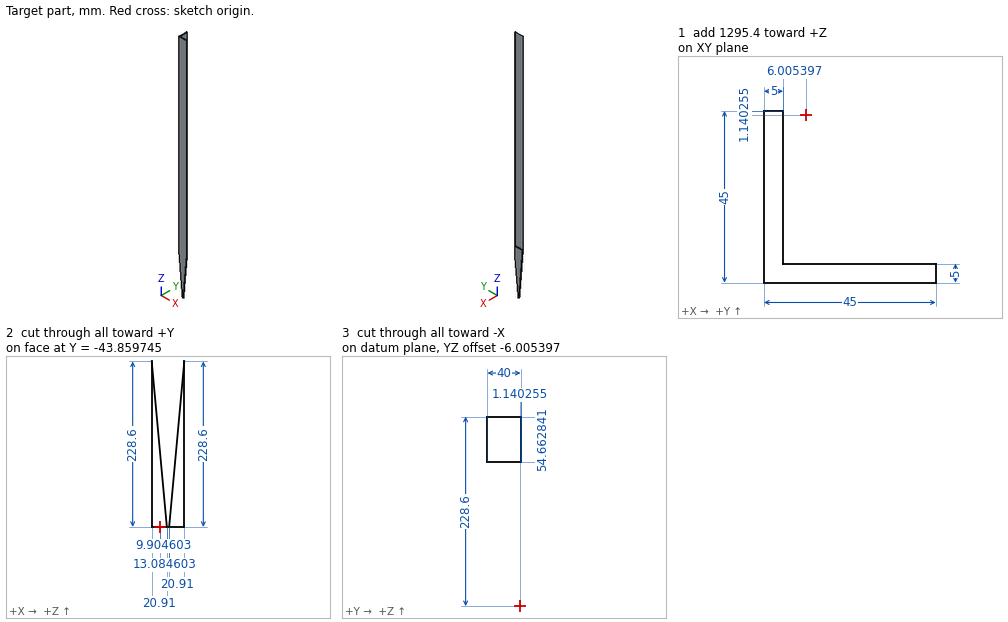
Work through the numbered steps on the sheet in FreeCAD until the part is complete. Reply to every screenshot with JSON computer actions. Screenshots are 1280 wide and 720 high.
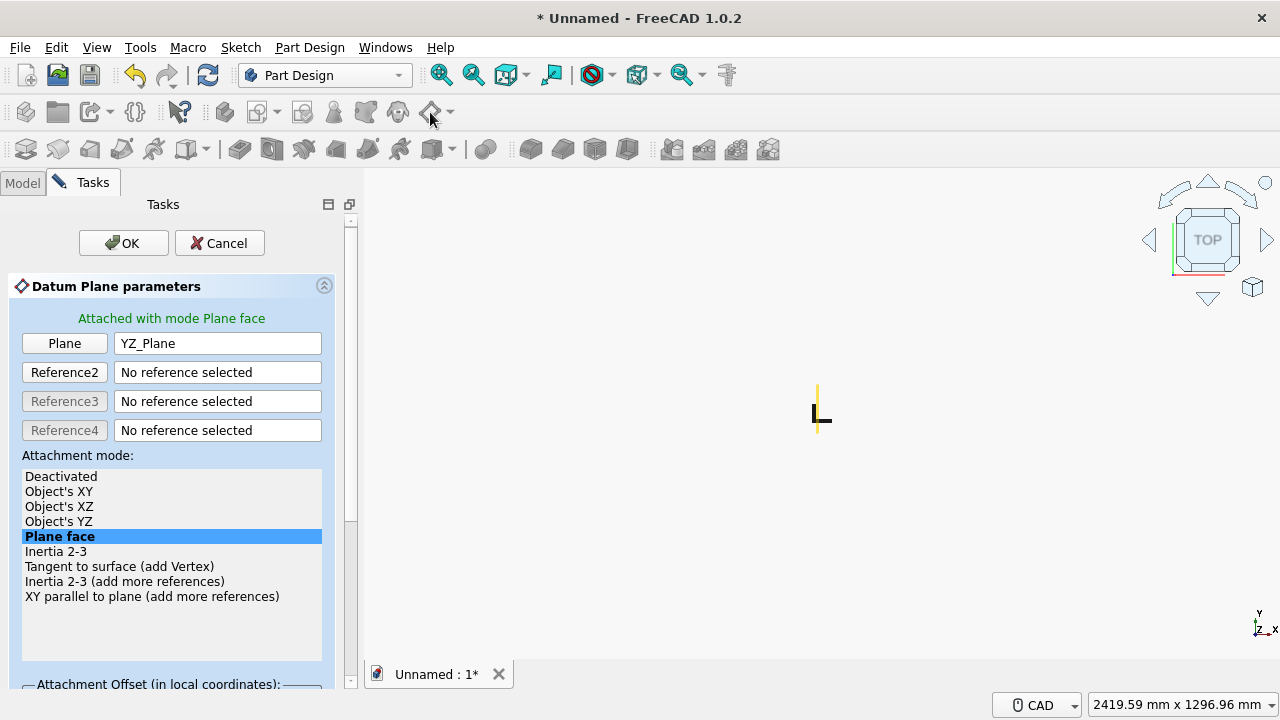
{"action": "scroll", "coordinate": [351, 451], "scroll_direction": "down", "scroll_amount": 3}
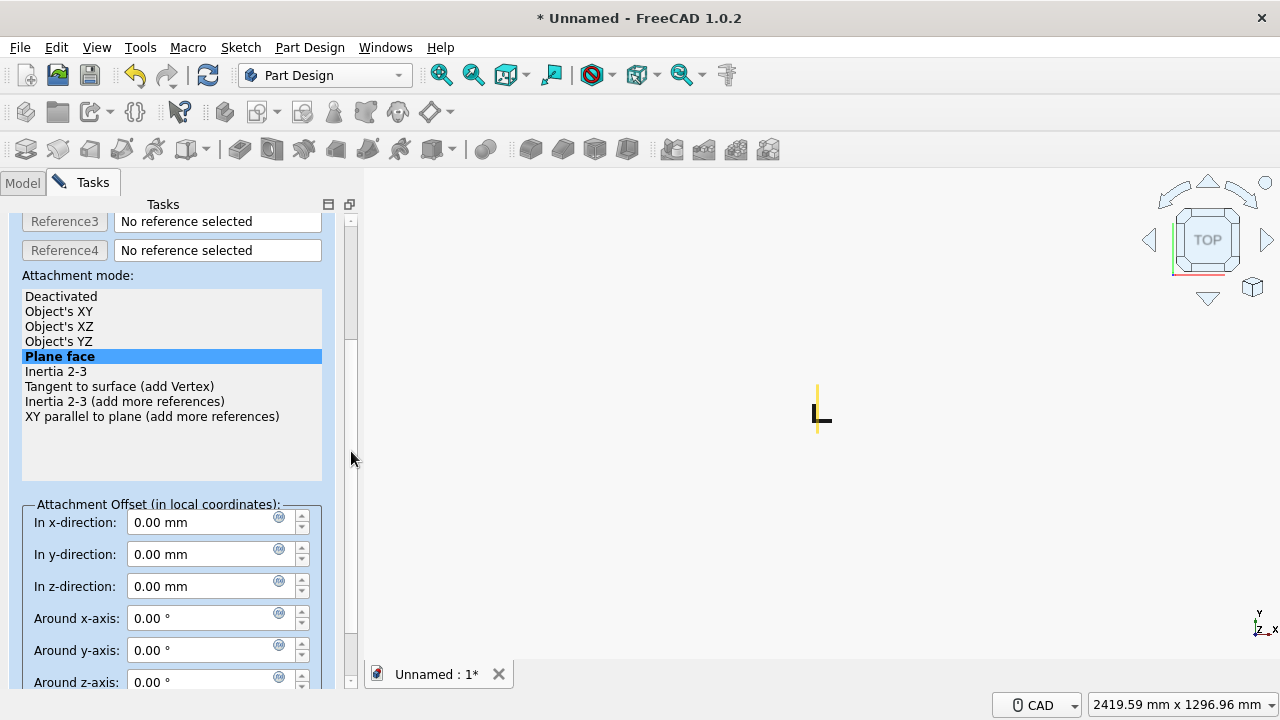
{"action": "triple_click", "coordinate": [210, 586]}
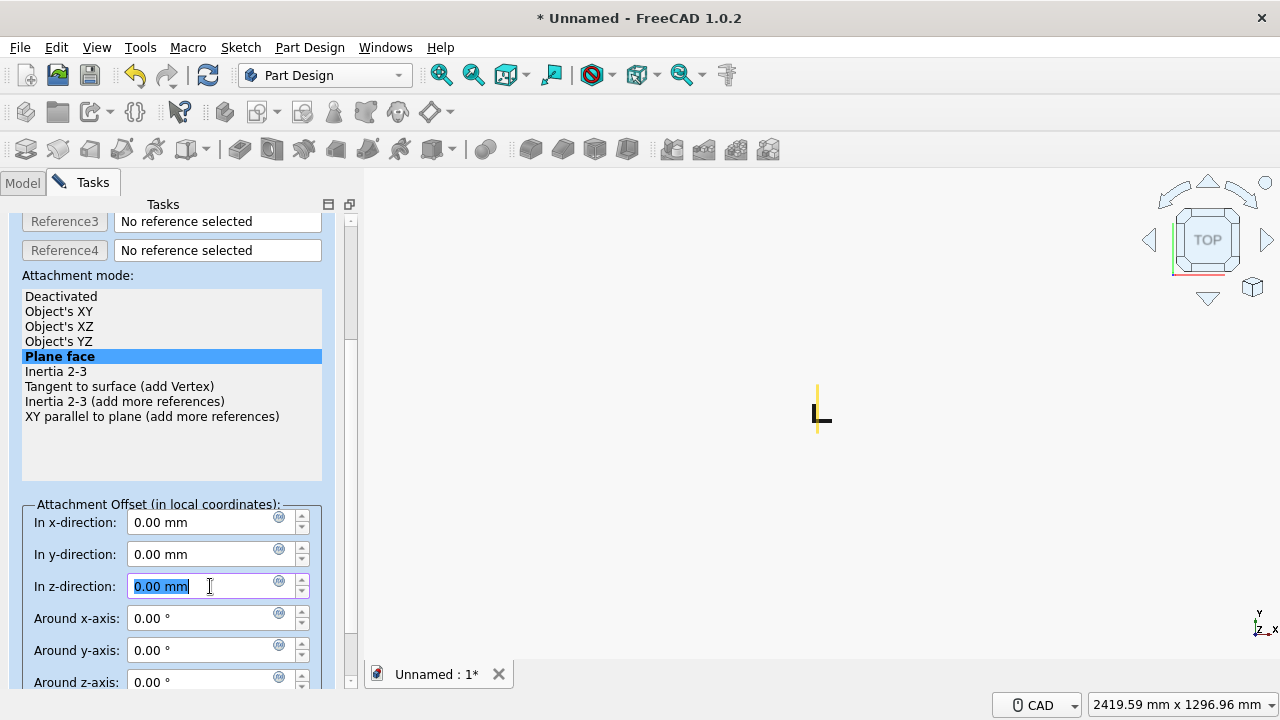
{"action": "type", "text": "-6.005397"}
{"action": "key", "text": "Tab"}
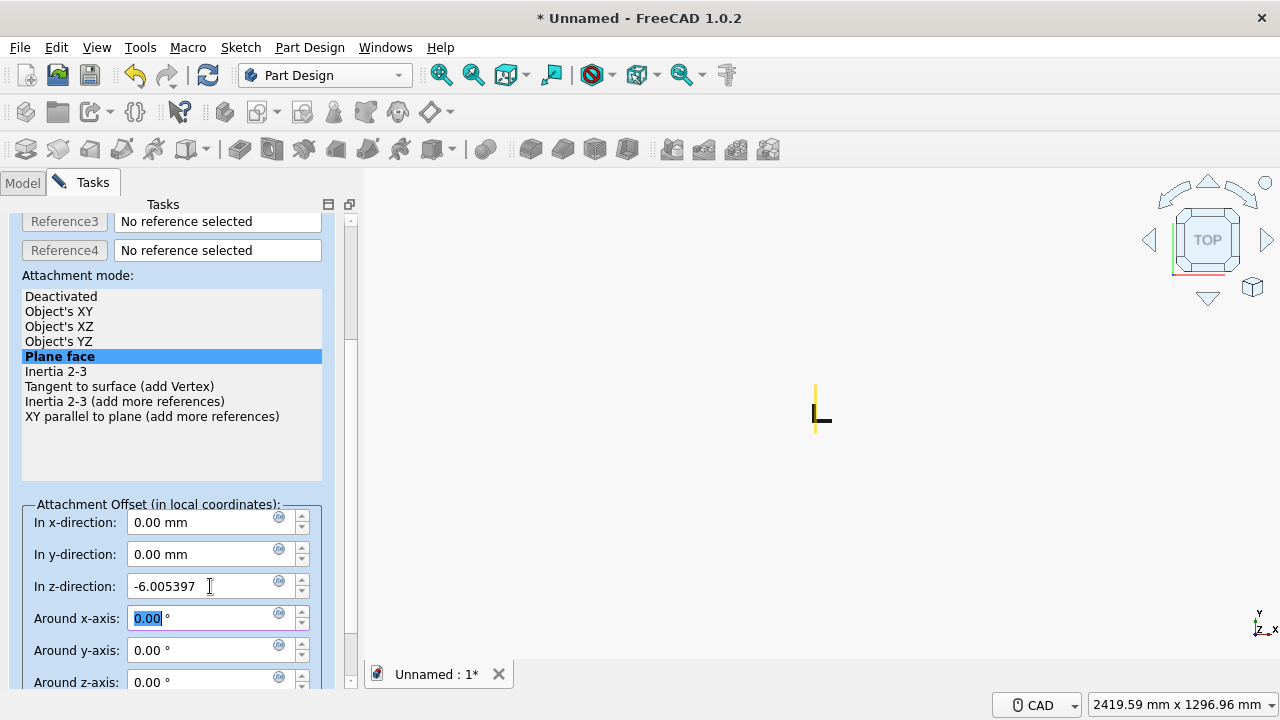
{"action": "scroll", "coordinate": [351, 451], "scroll_direction": "up", "scroll_amount": 4}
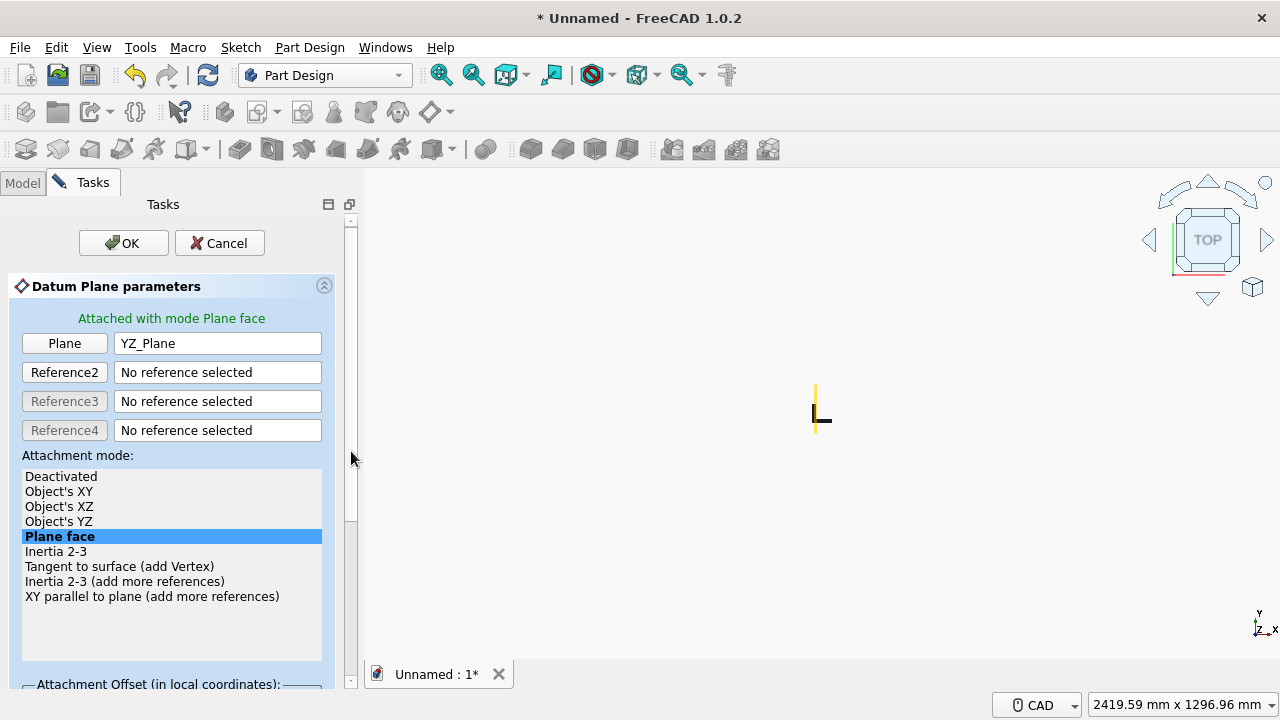
{"action": "left_click", "coordinate": [124, 243]}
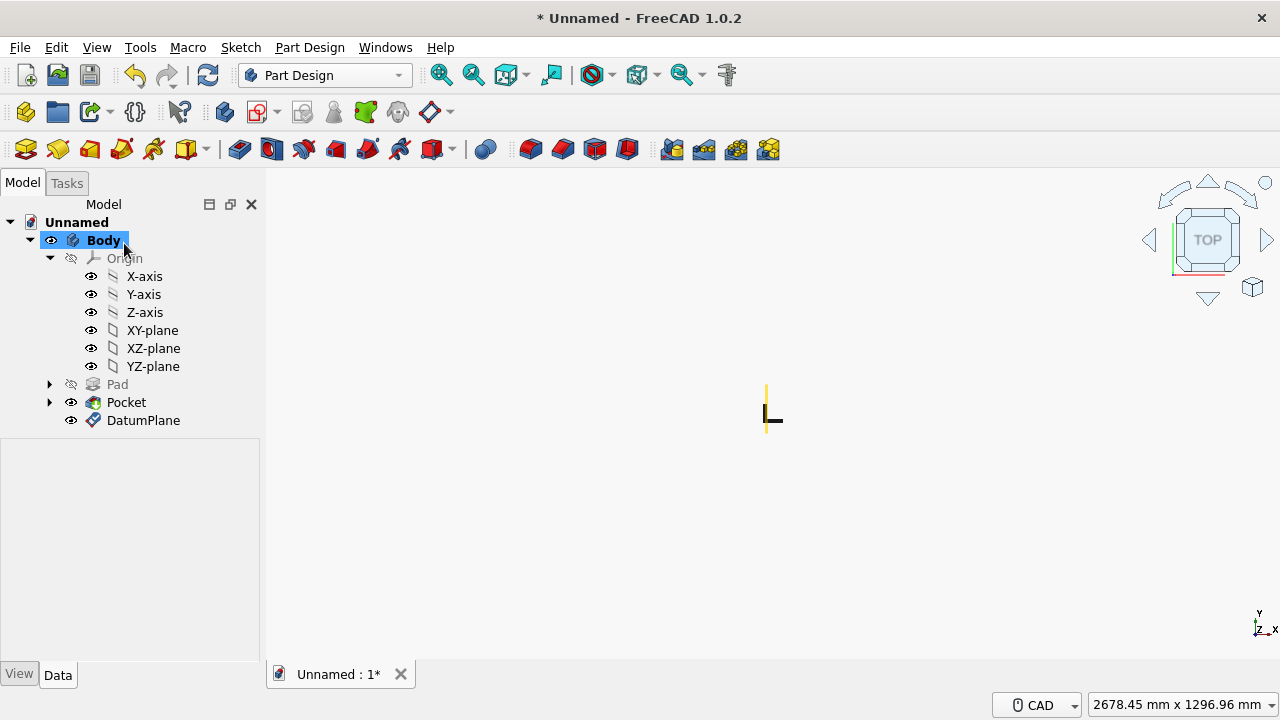
{"action": "left_click", "coordinate": [116, 420]}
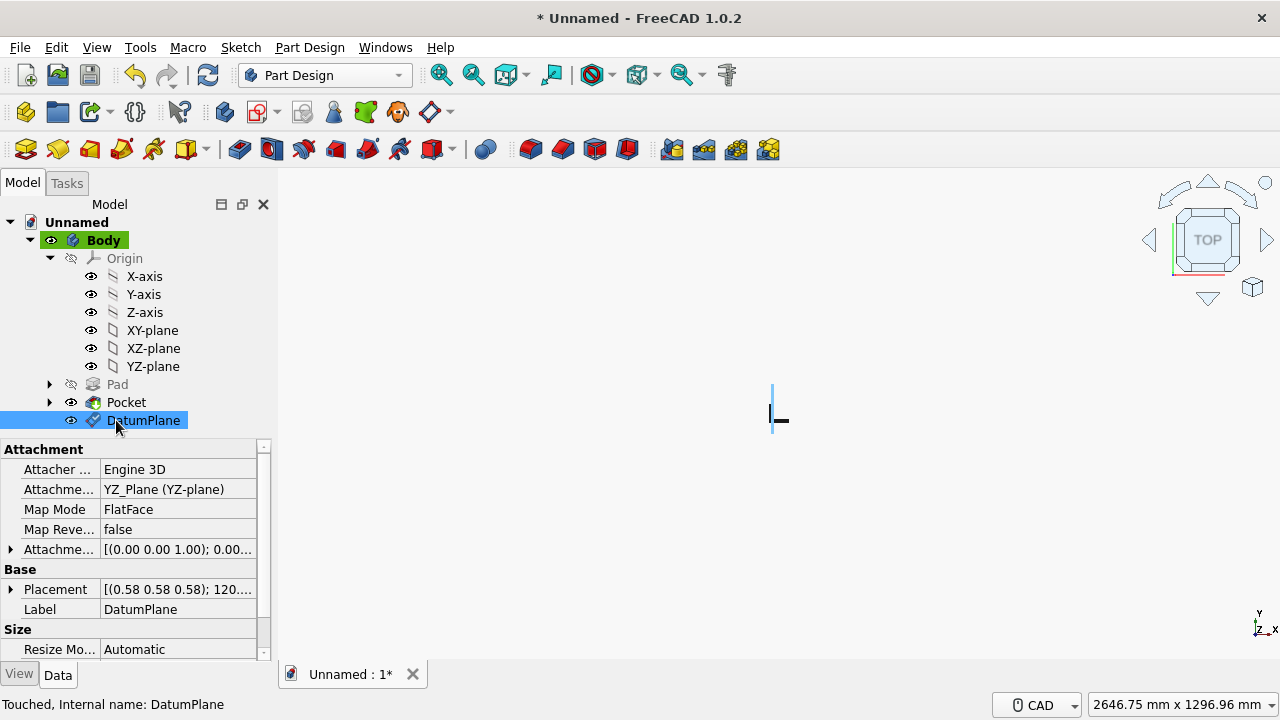
{"action": "left_click", "coordinate": [258, 112]}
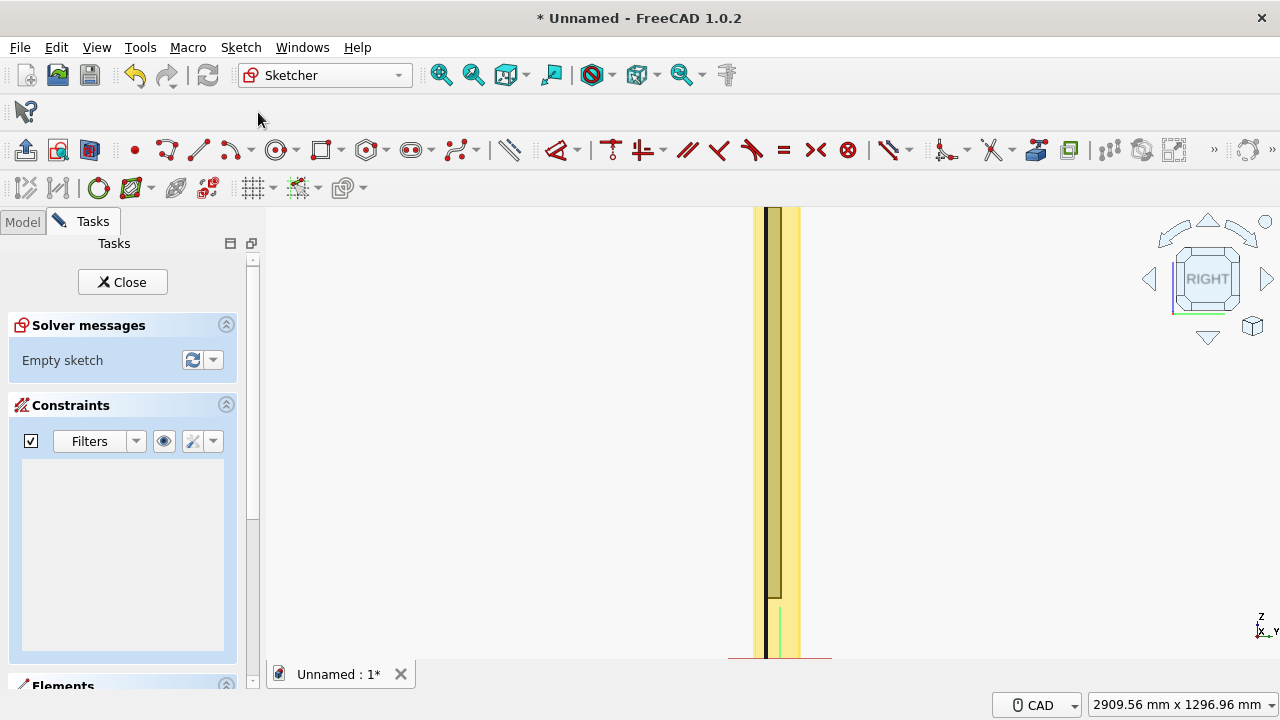
{"action": "key", "text": "q s"}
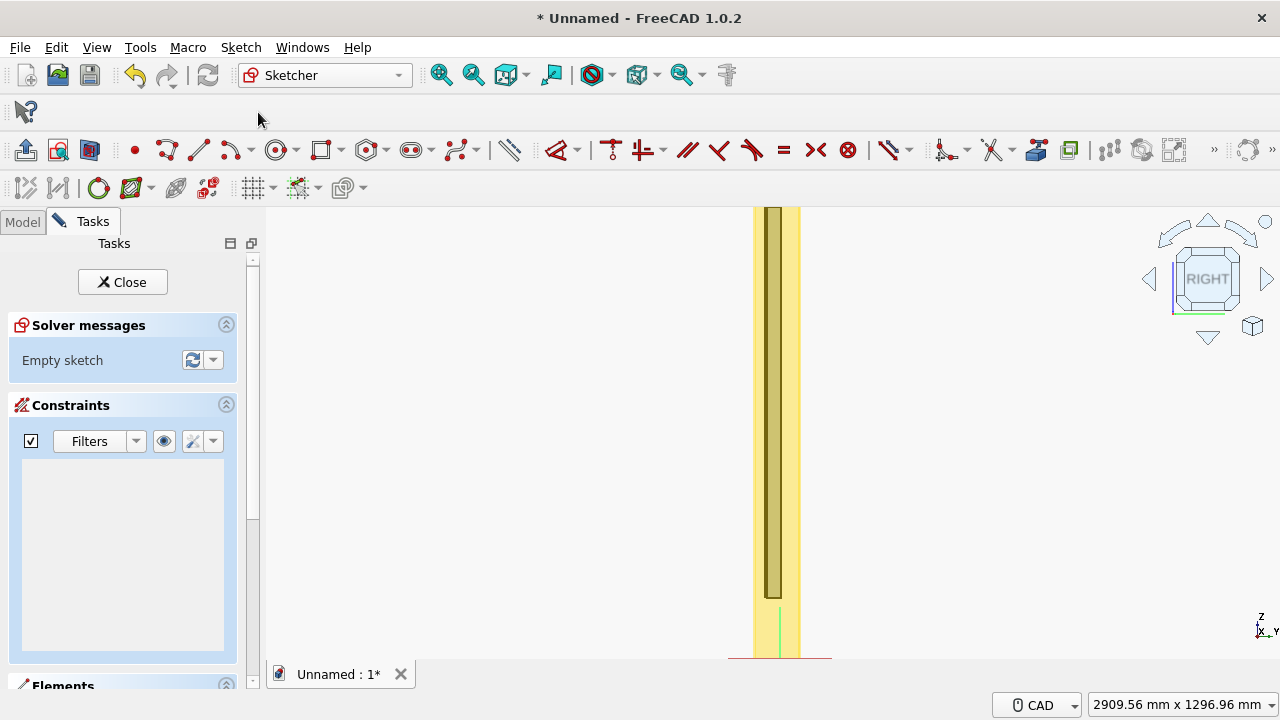
{"action": "scroll", "coordinate": [779, 601], "scroll_direction": "up", "scroll_amount": 13}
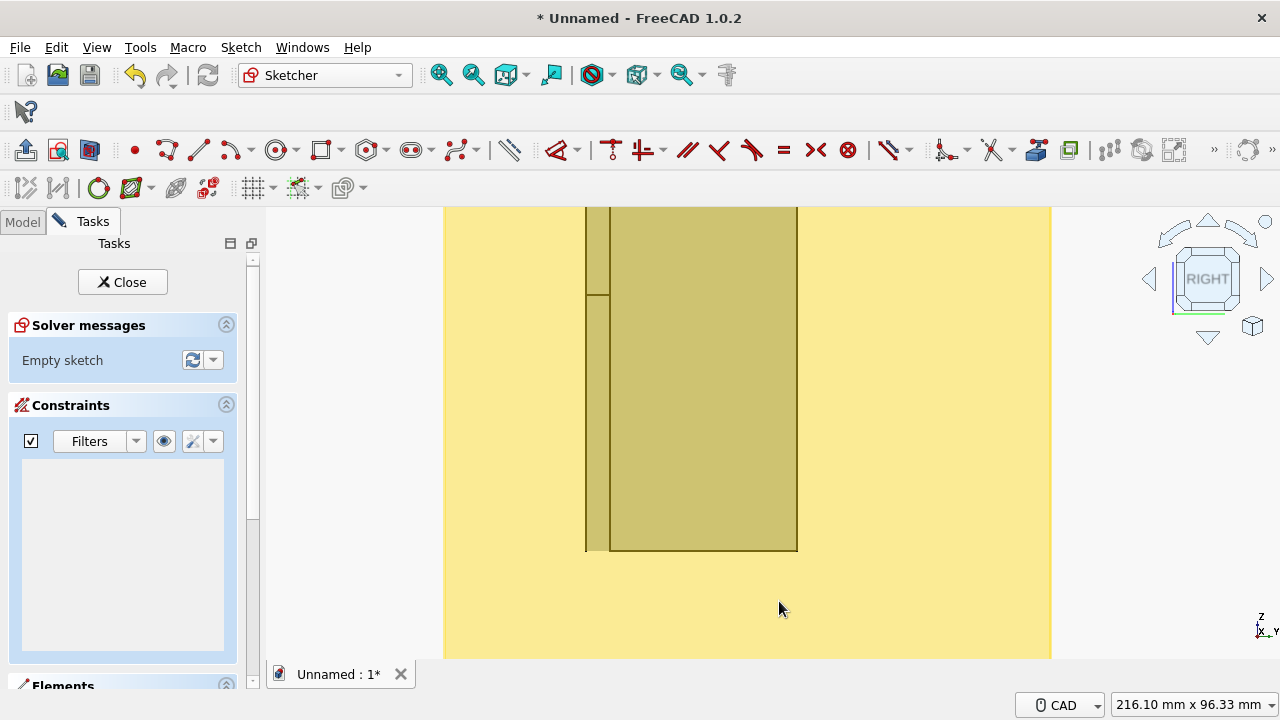
{"action": "left_click", "coordinate": [322, 150]}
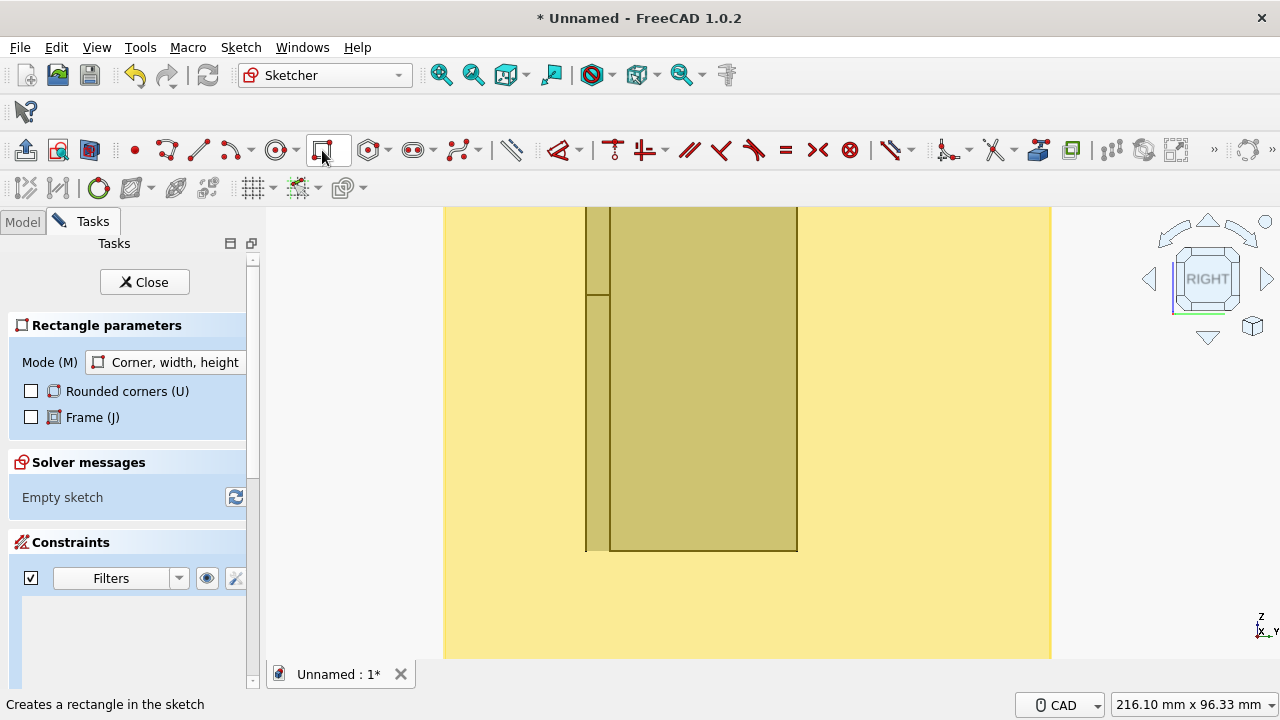
{"action": "left_click", "coordinate": [610, 295]}